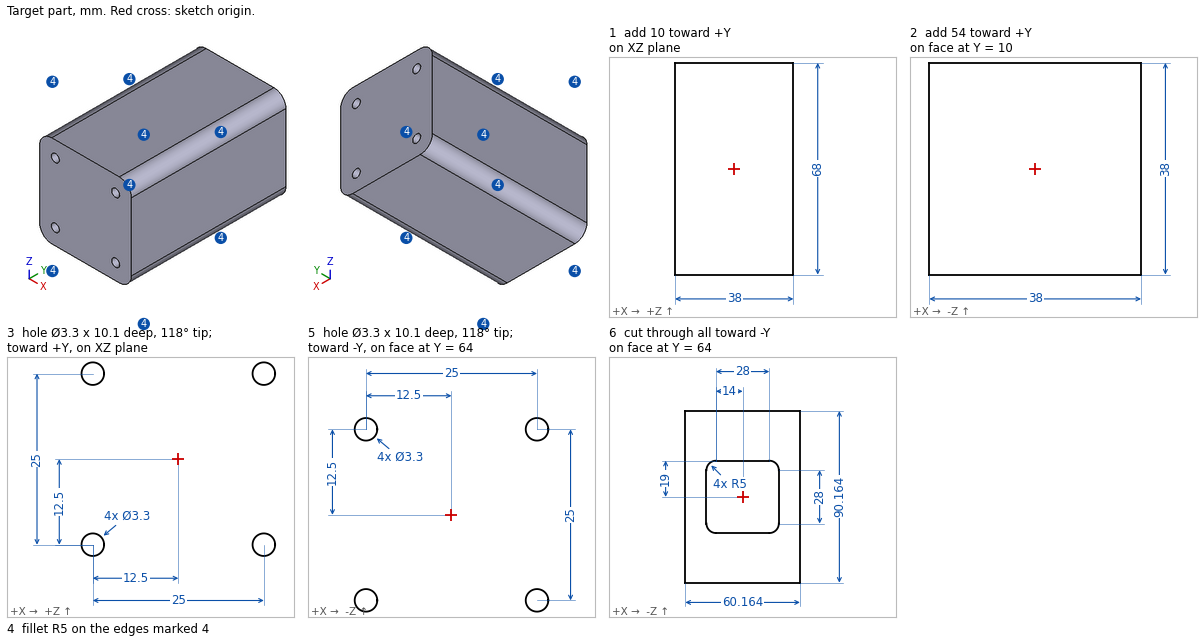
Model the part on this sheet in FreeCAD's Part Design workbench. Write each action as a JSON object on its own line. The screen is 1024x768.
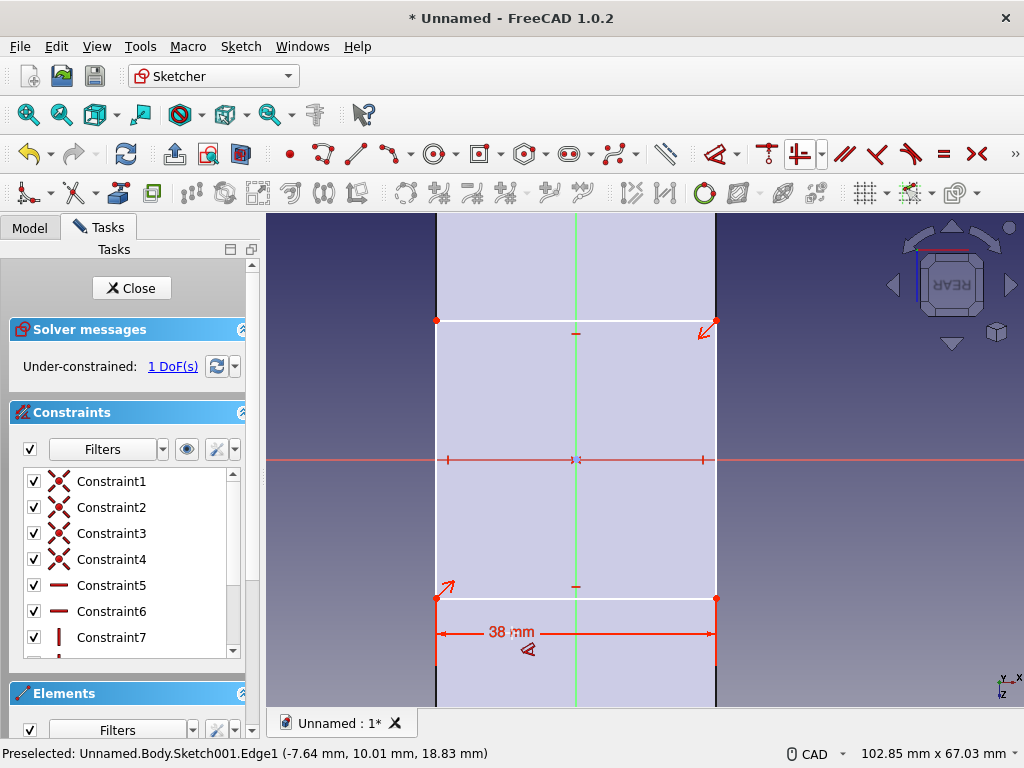
{"action": "left_click", "coordinate": [716, 515]}
{"action": "left_click", "coordinate": [750, 396]}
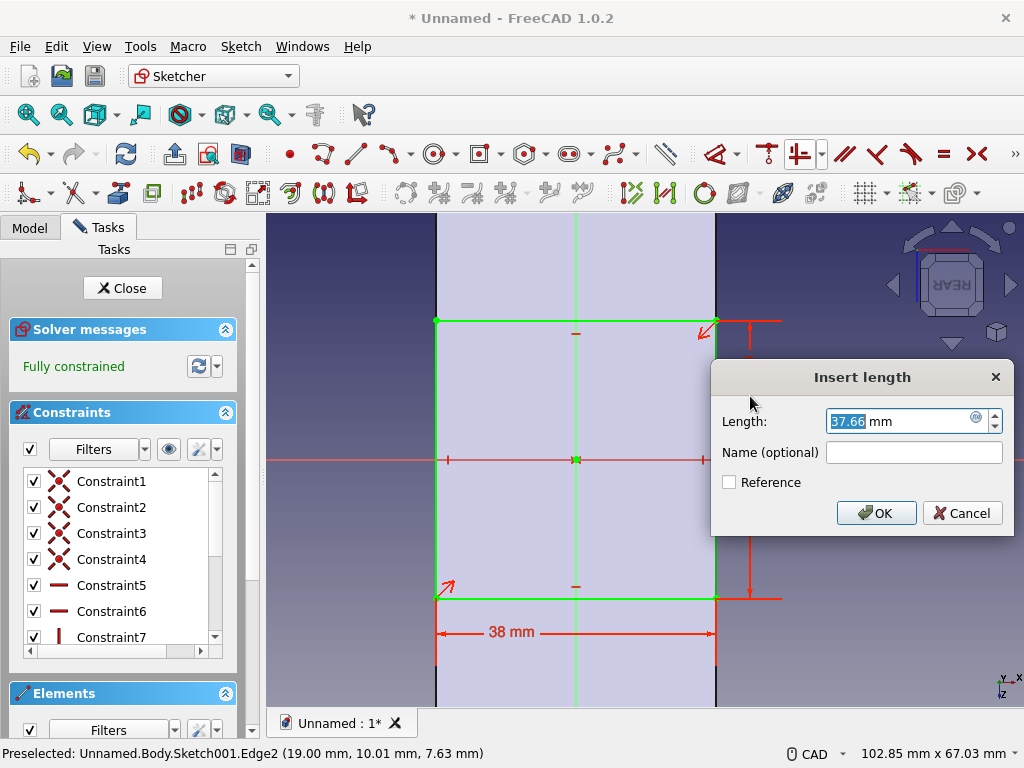
{"action": "type", "text": "38"}
{"action": "key", "text": "Return"}
{"action": "key", "text": "Escape"}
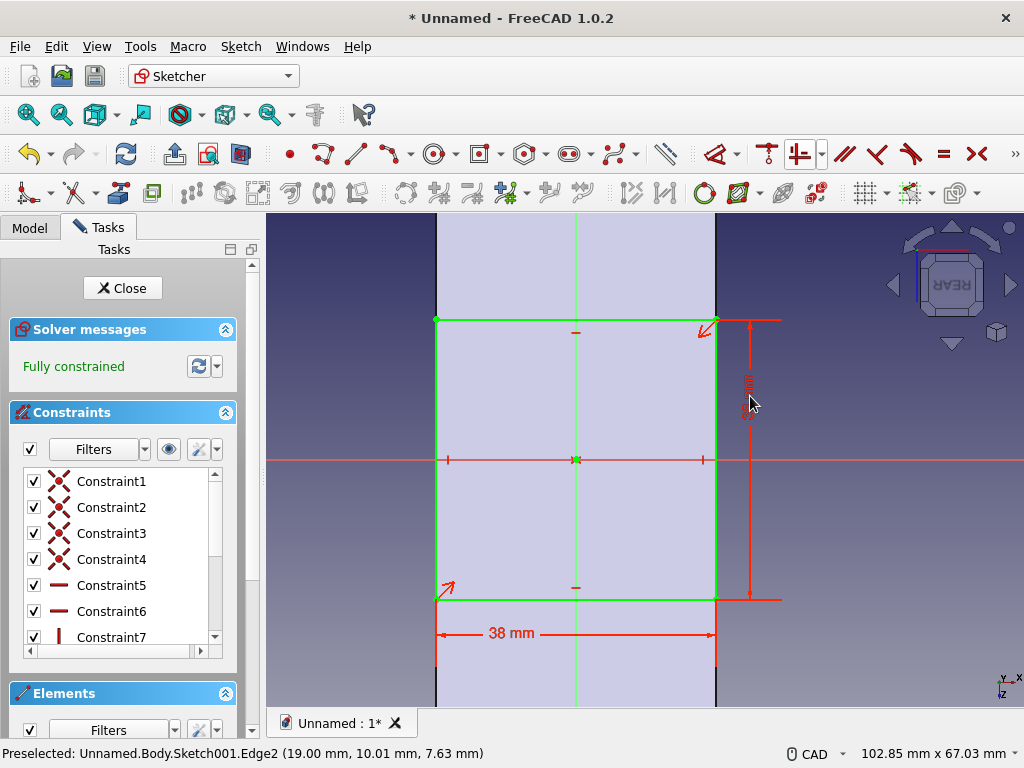
{"action": "left_click", "coordinate": [123, 288]}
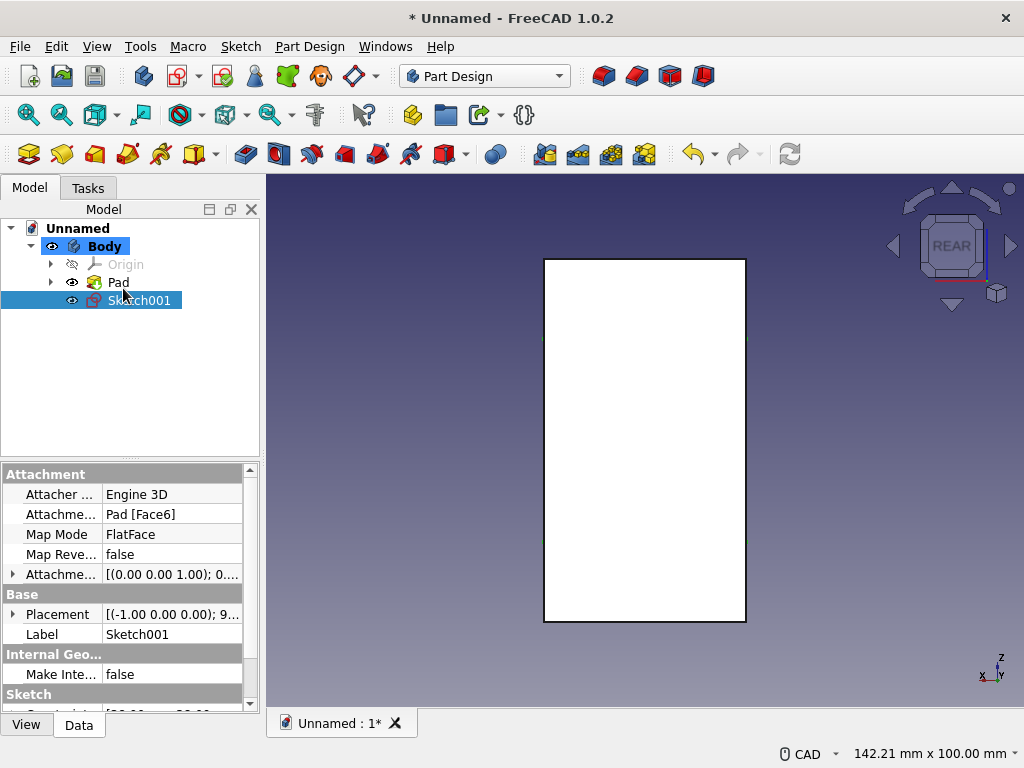
{"action": "left_click", "coordinate": [29, 154]}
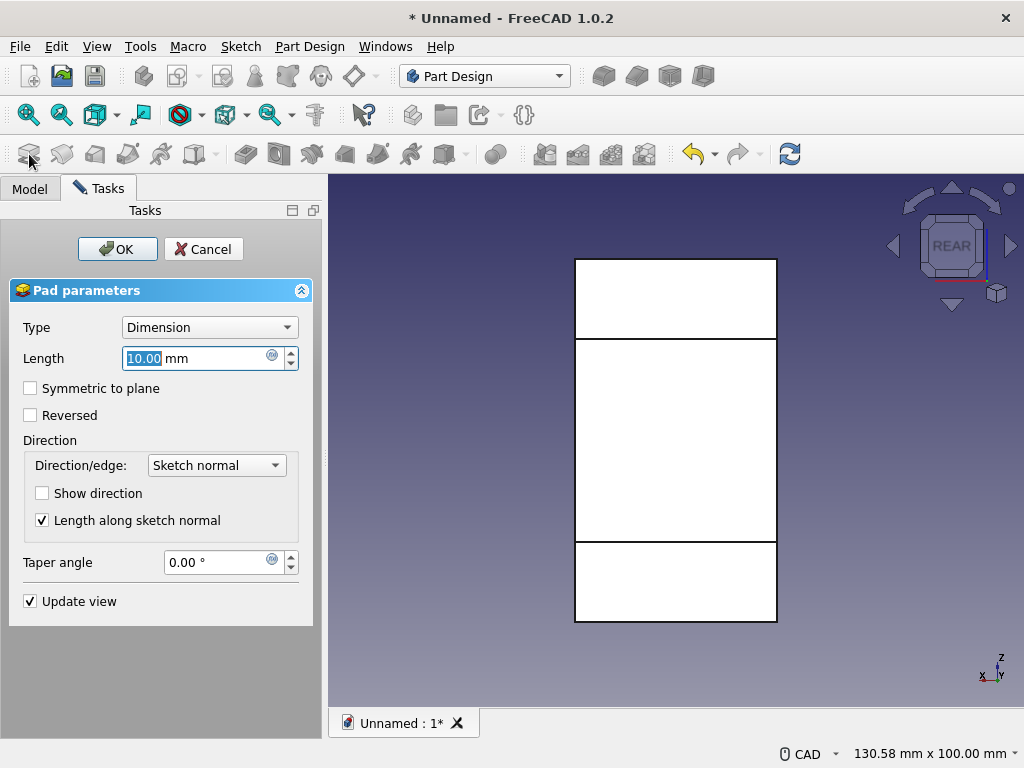
{"action": "type", "text": "54"}
{"action": "key", "text": "Tab"}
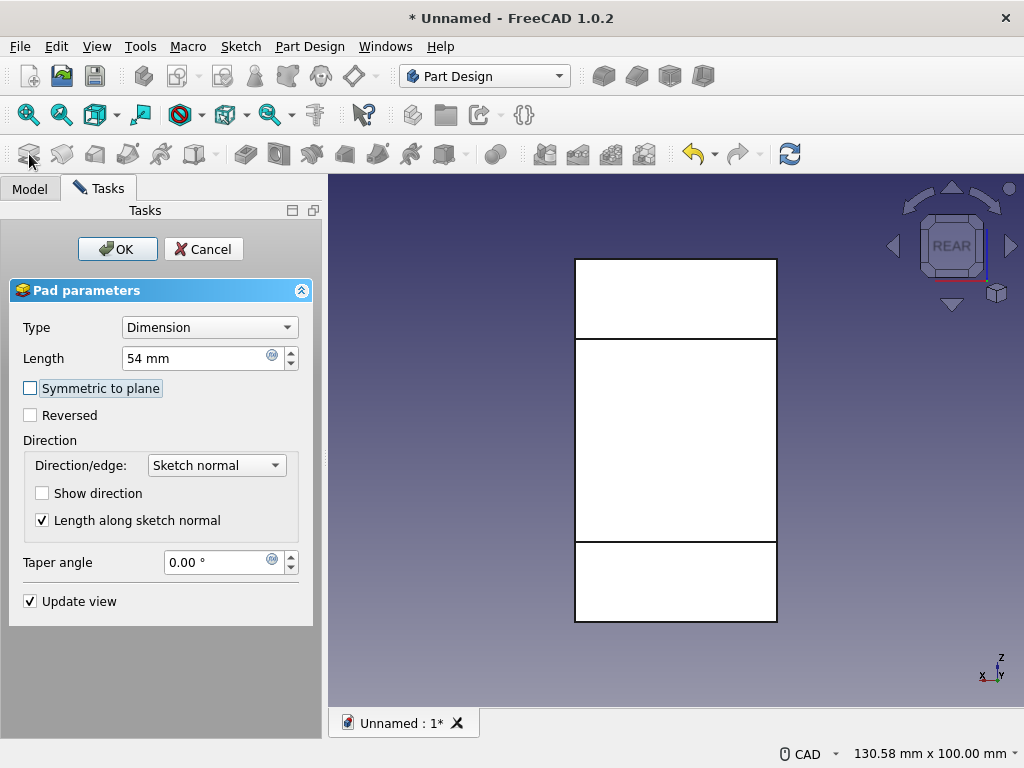
{"action": "left_click", "coordinate": [118, 249]}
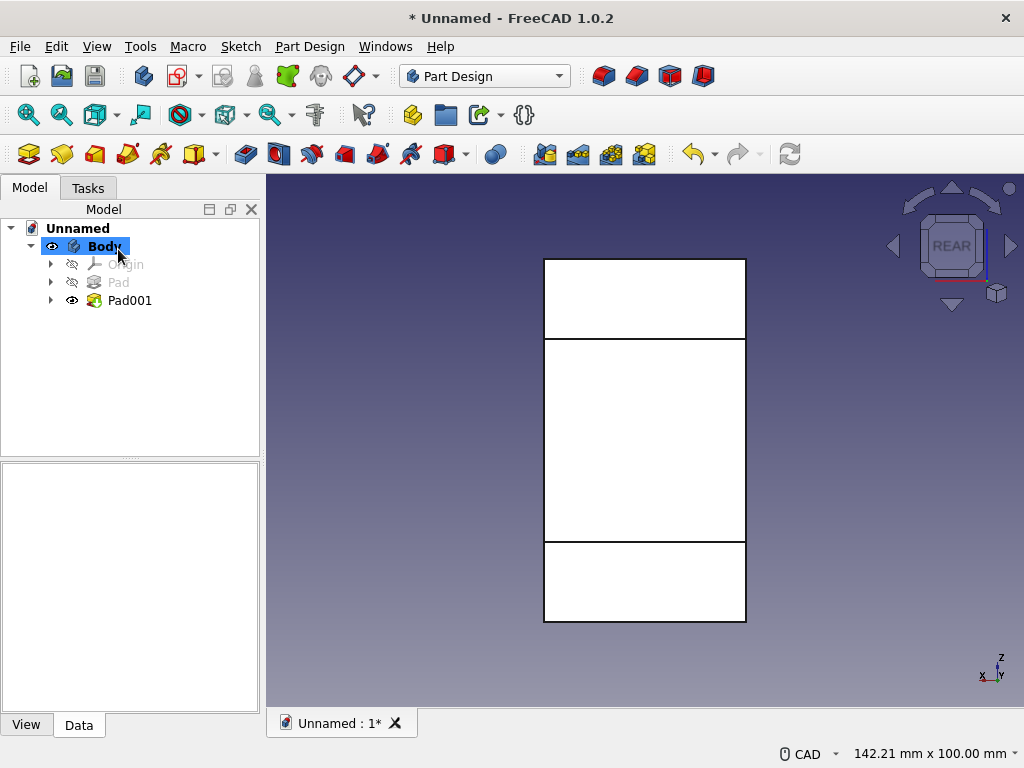
{"action": "left_click", "coordinate": [176, 76]}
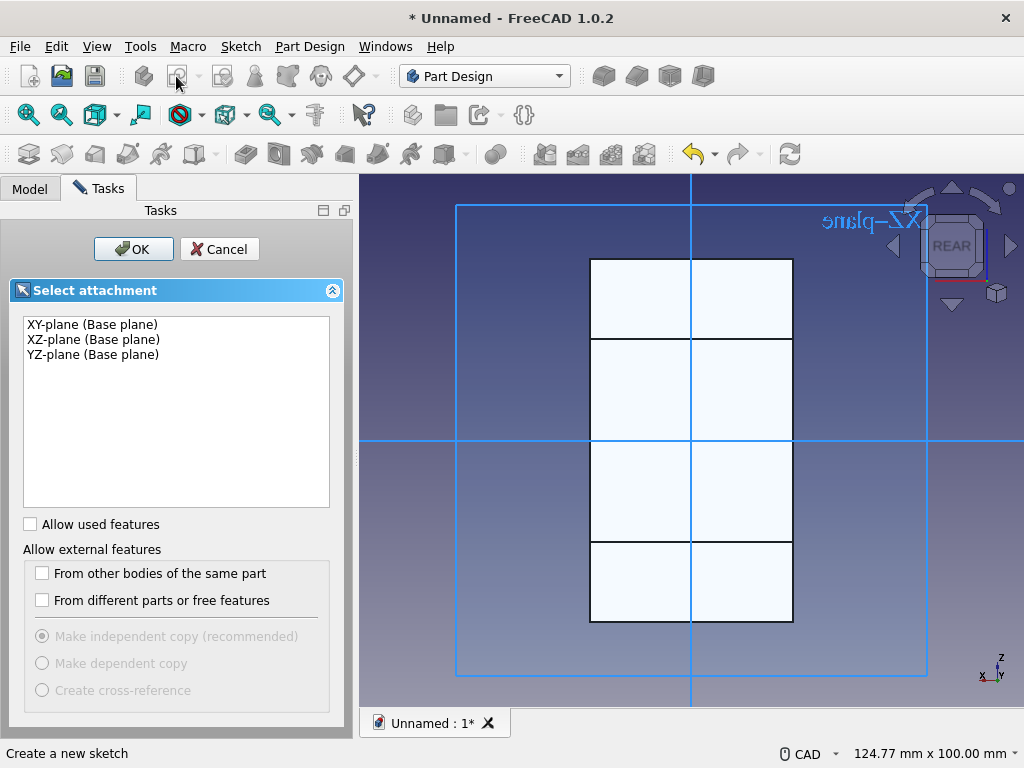
{"action": "left_click", "coordinate": [84, 340]}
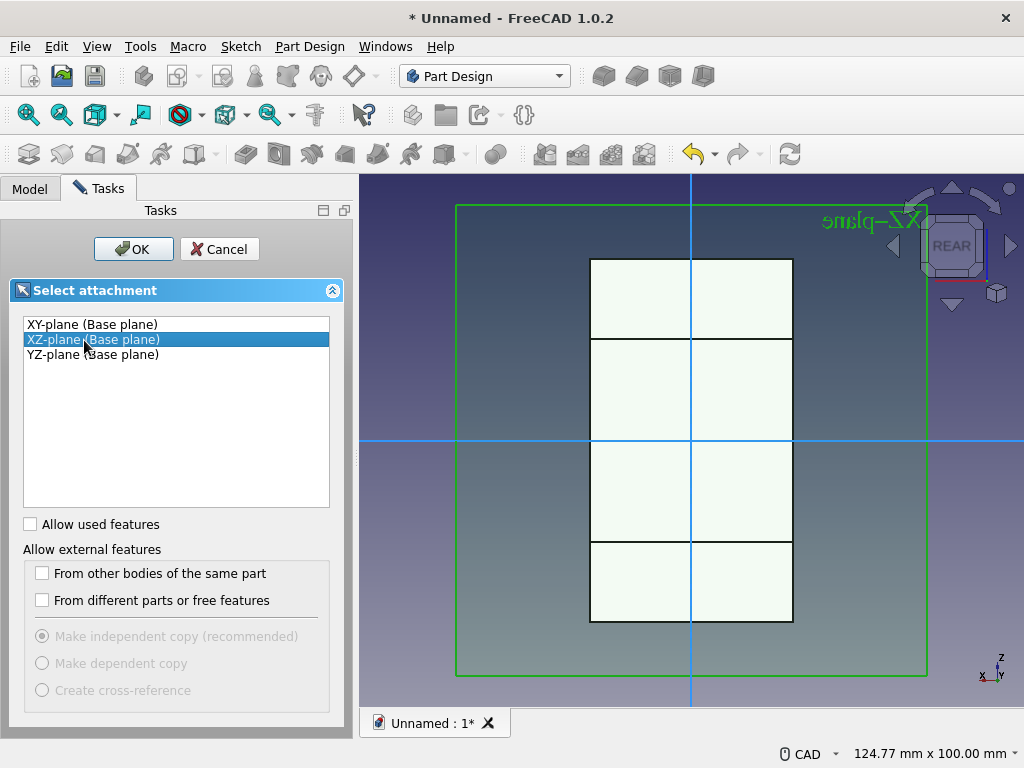
{"action": "left_click", "coordinate": [134, 249]}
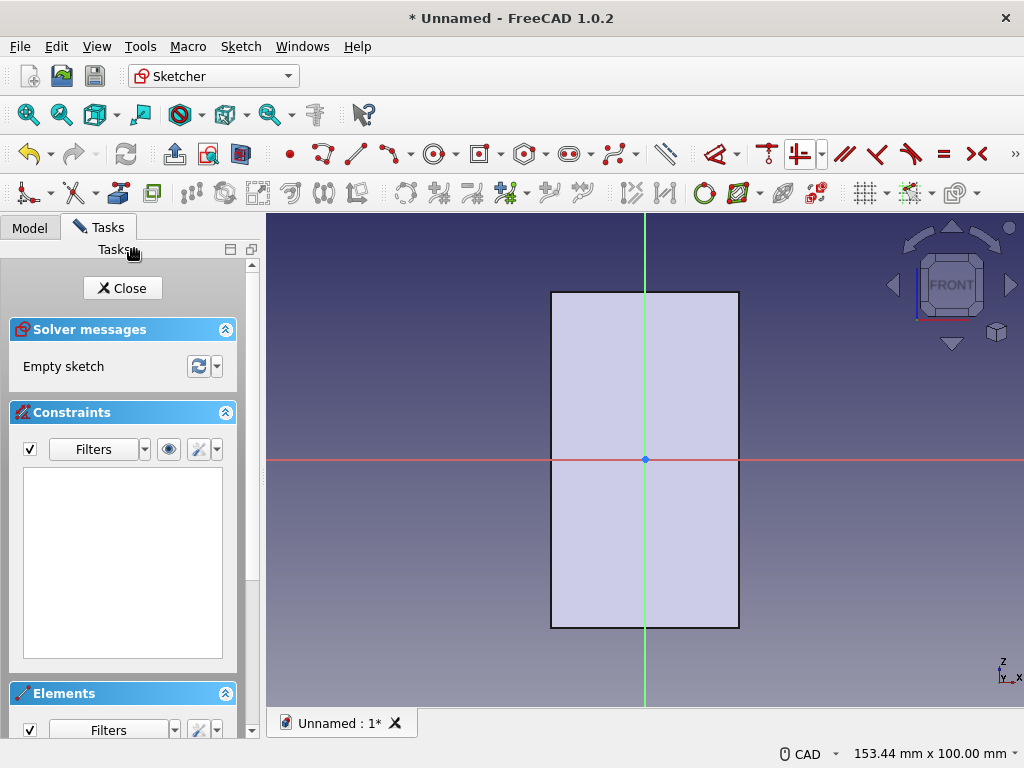
{"action": "scroll", "coordinate": [701, 460], "scroll_direction": "up", "scroll_amount": 4}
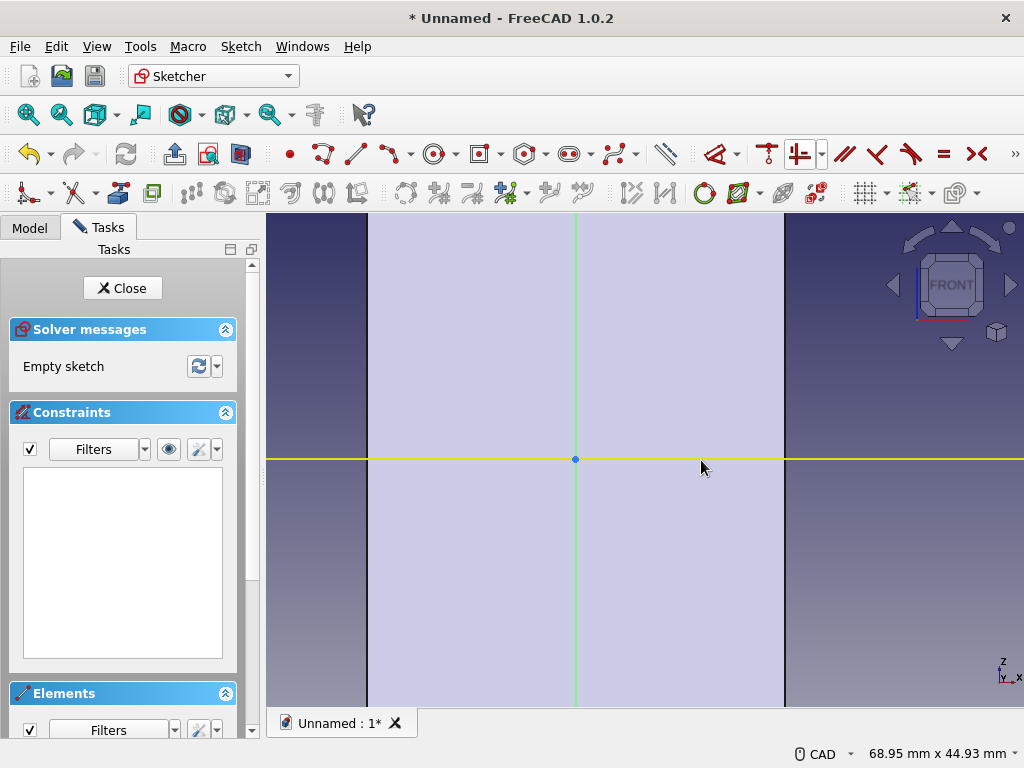
{"action": "left_click", "coordinate": [434, 154]}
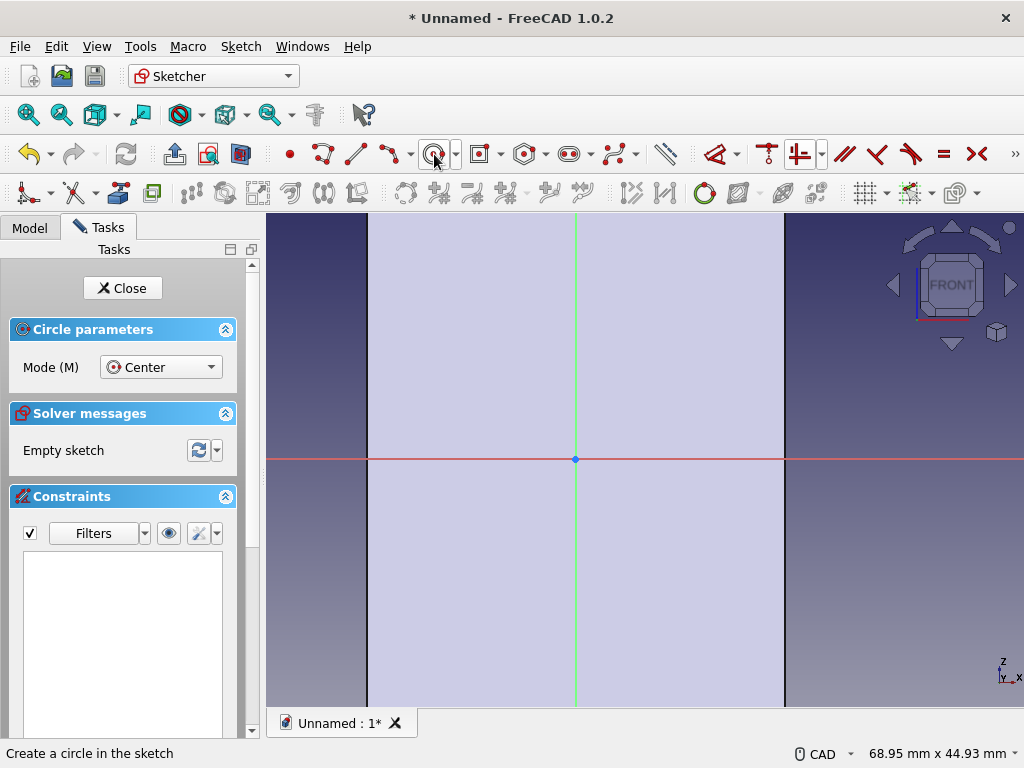
{"action": "scroll", "coordinate": [438, 597], "scroll_direction": "up", "scroll_amount": 2}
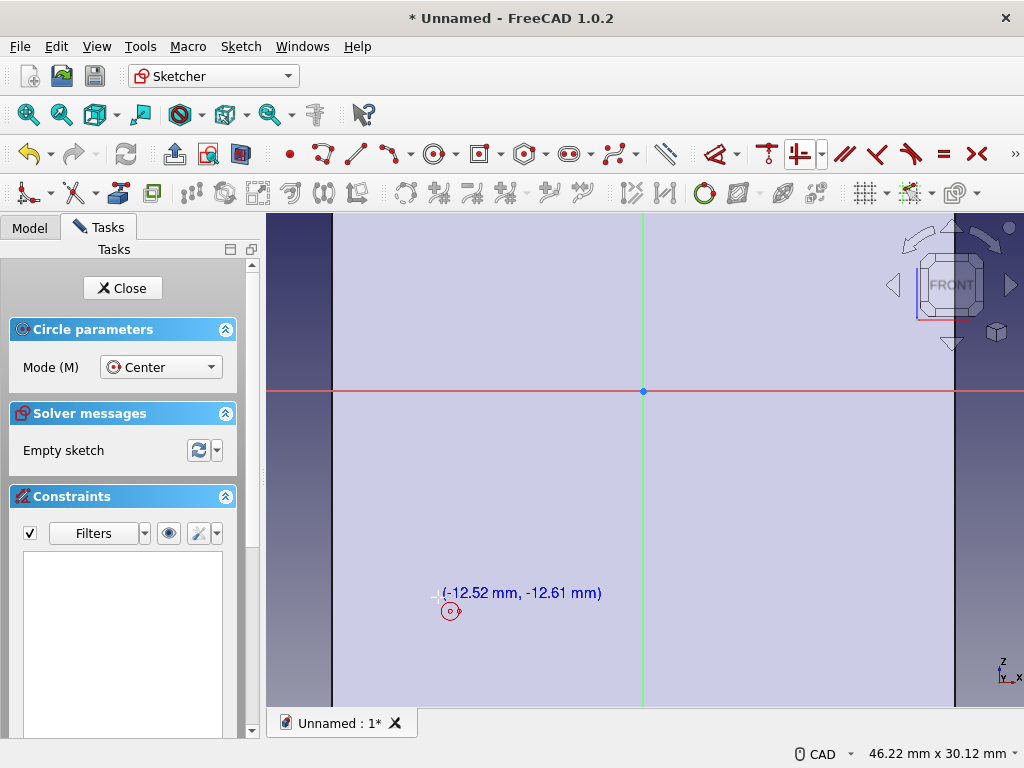
{"action": "left_click", "coordinate": [438, 596]}
{"action": "left_click", "coordinate": [457, 577]}